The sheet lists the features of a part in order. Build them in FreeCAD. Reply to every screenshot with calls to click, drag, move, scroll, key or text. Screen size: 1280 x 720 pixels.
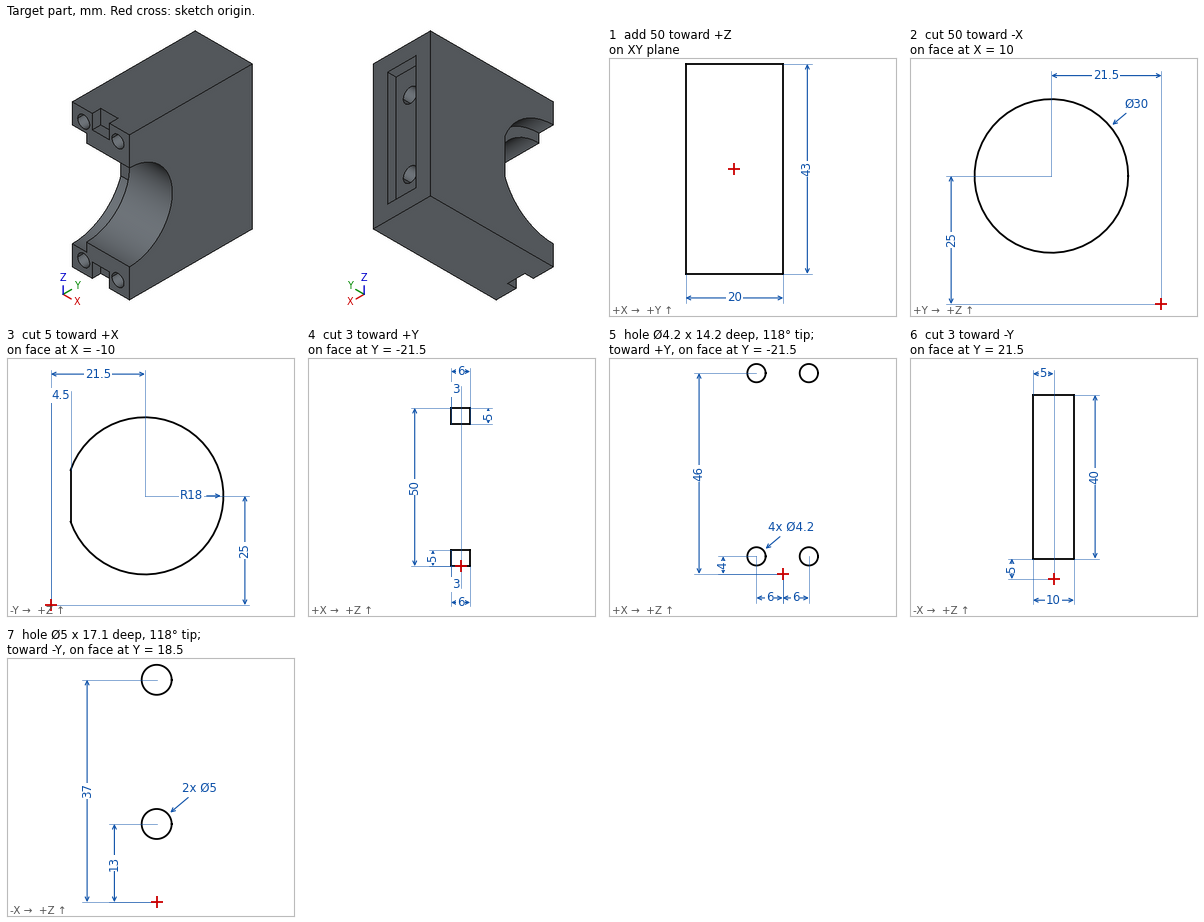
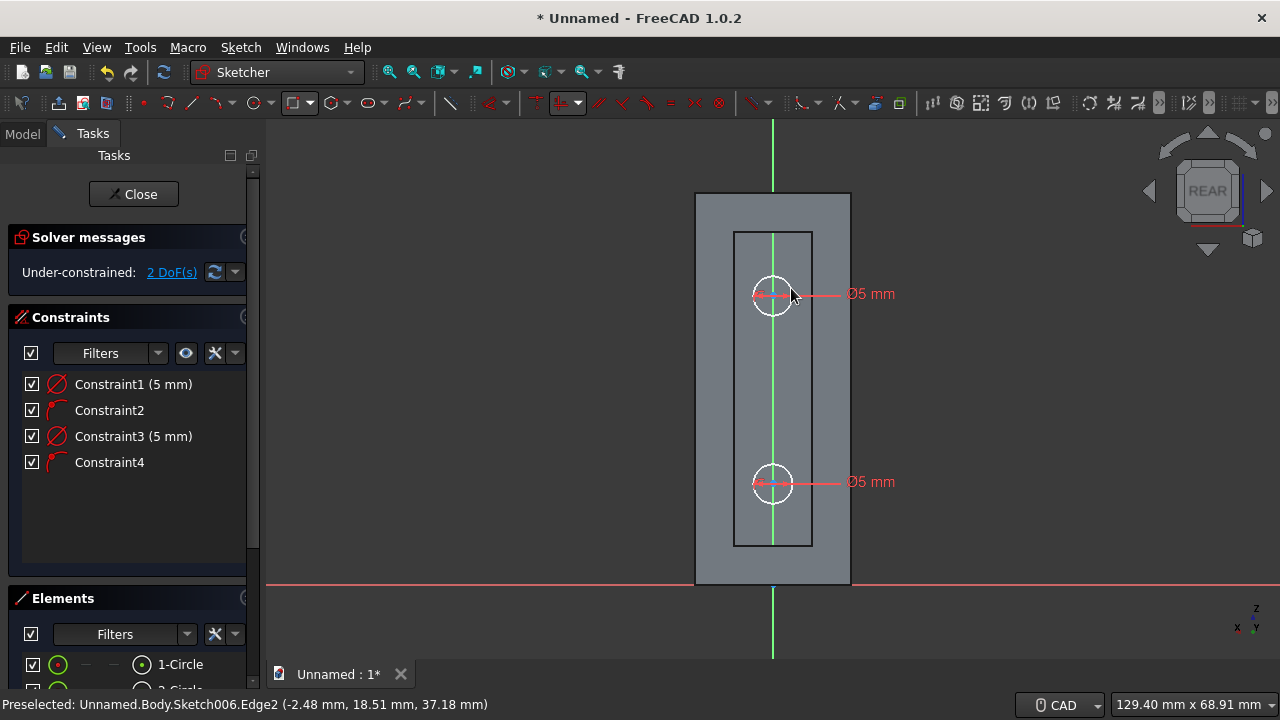
click(490, 104)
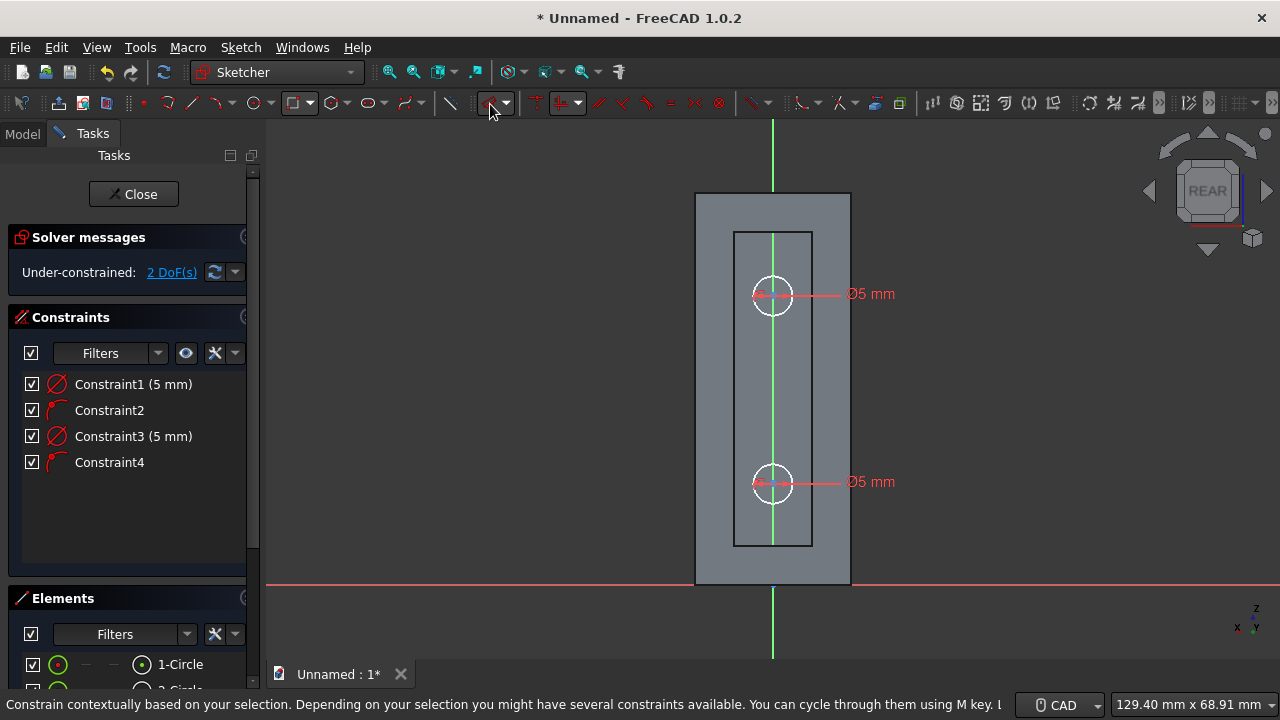
click(773, 484)
click(807, 534)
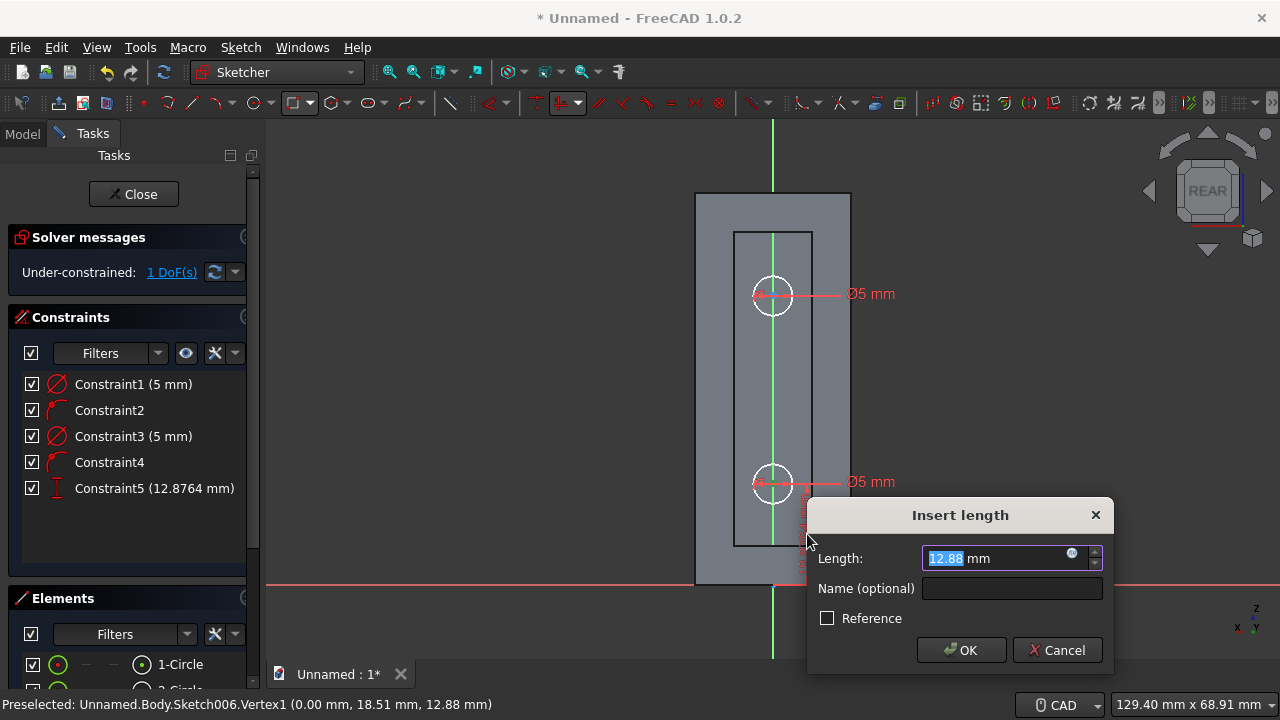
text(13)
key(Return)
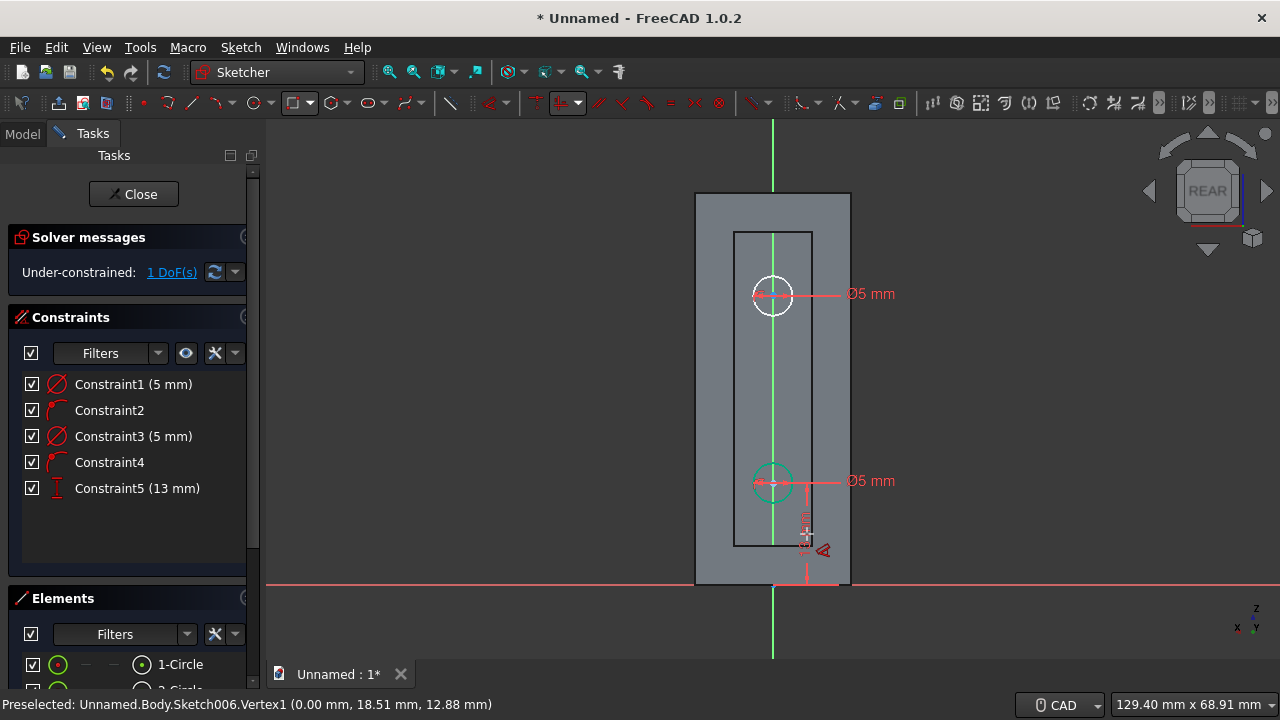
click(773, 296)
click(807, 440)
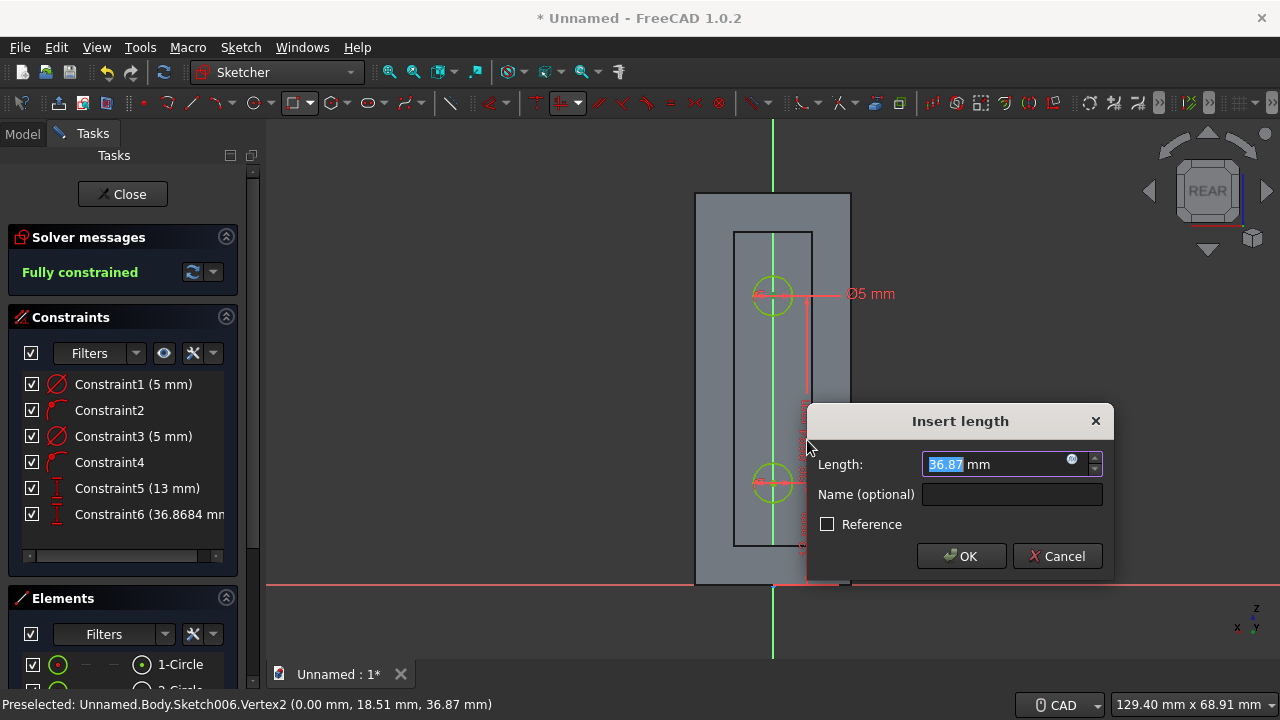
text(37)
key(Return)
key(Escape)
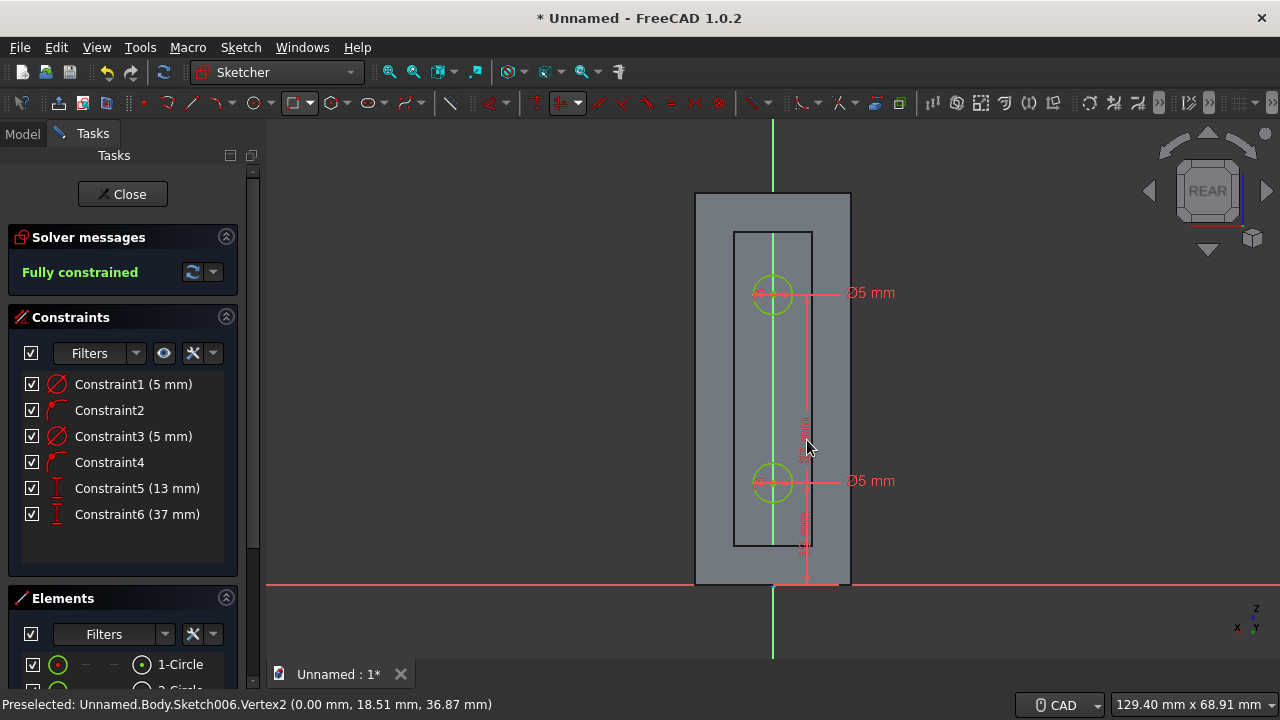
click(123, 194)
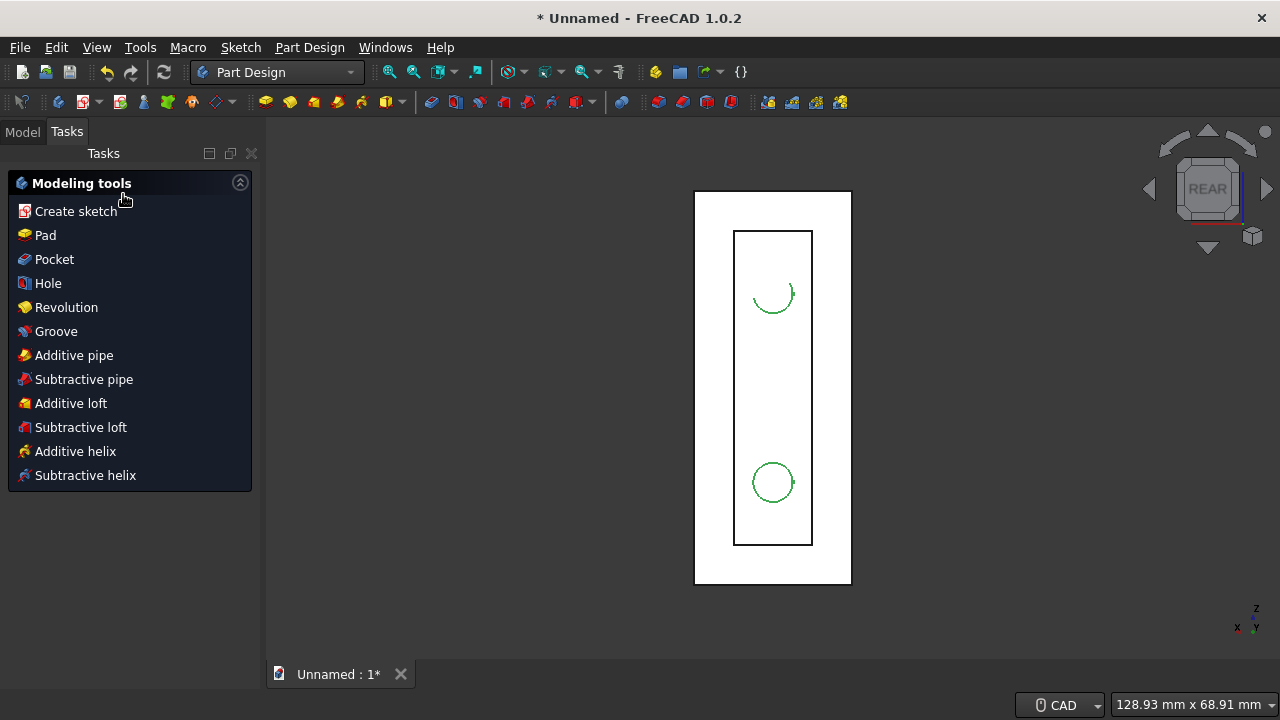
click(456, 102)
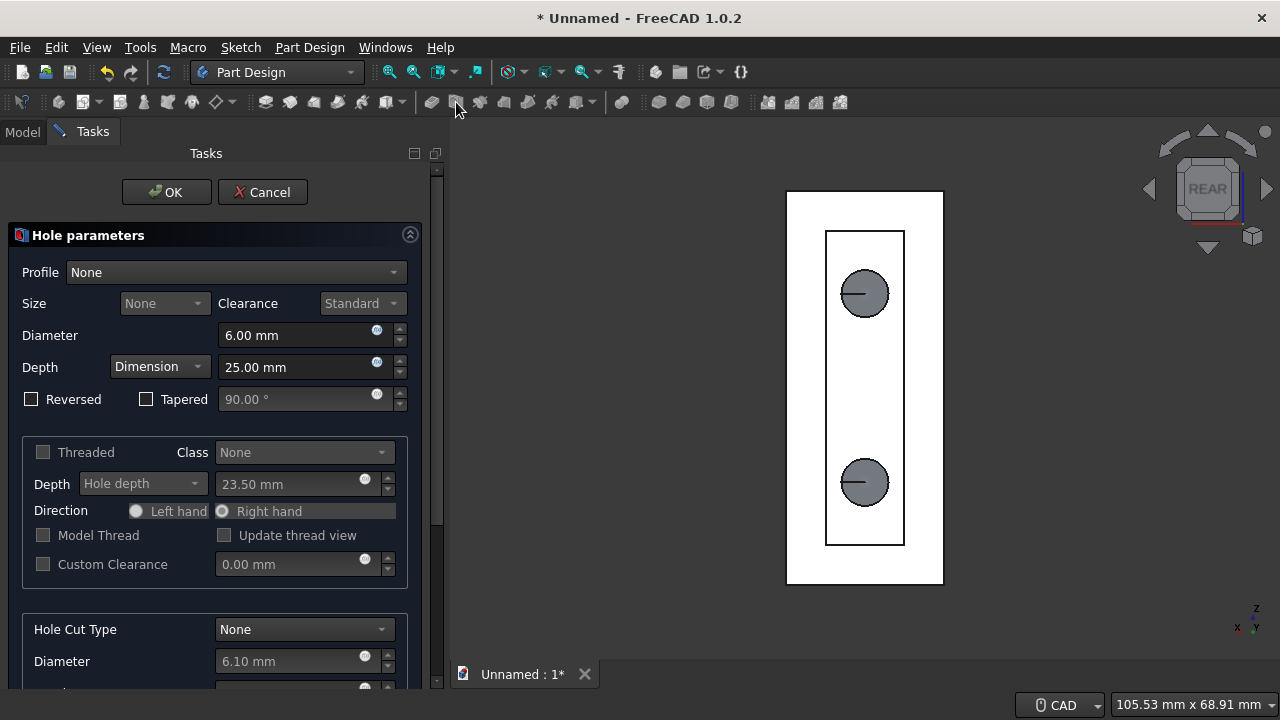
triple_click(305, 335)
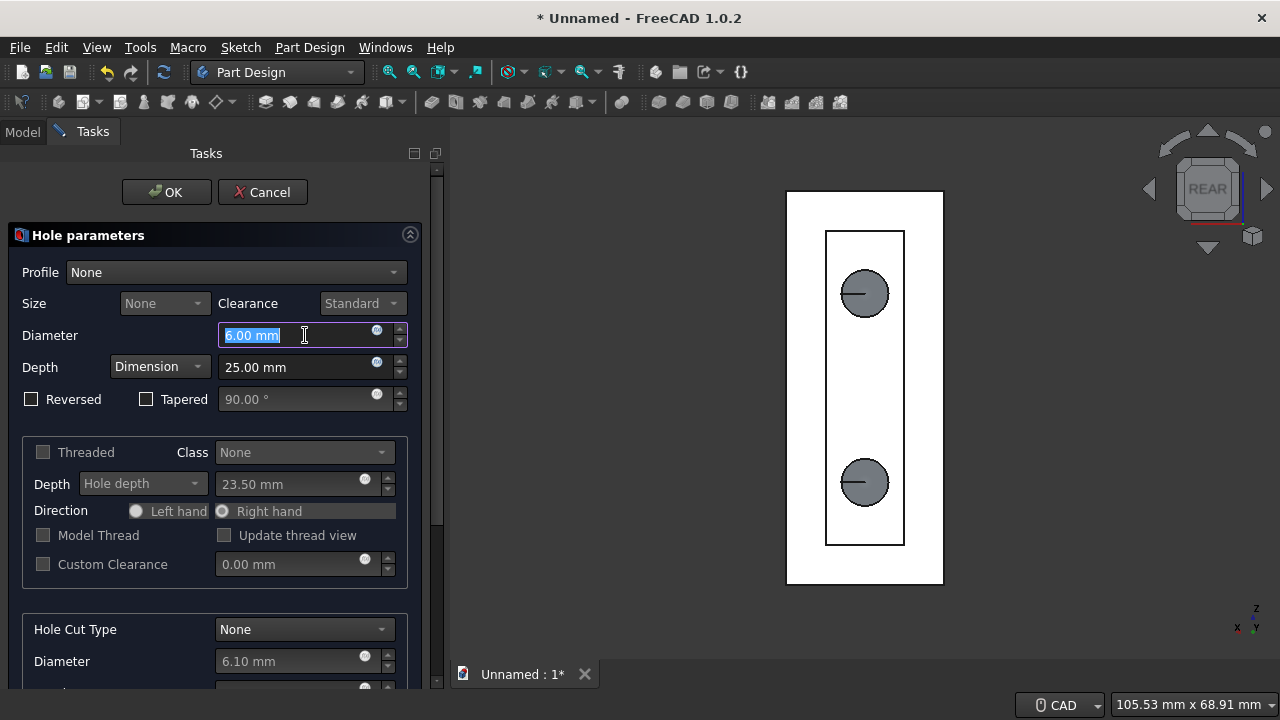
text(5)
key(Tab)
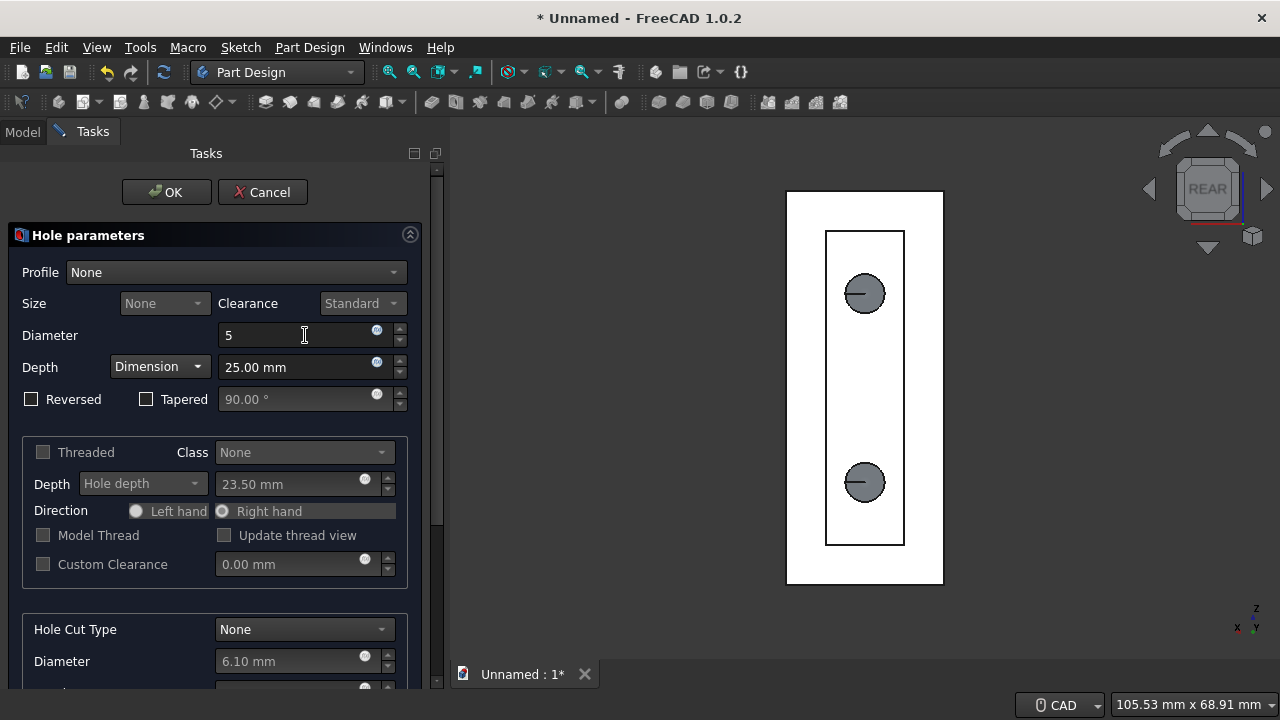
triple_click(305, 367)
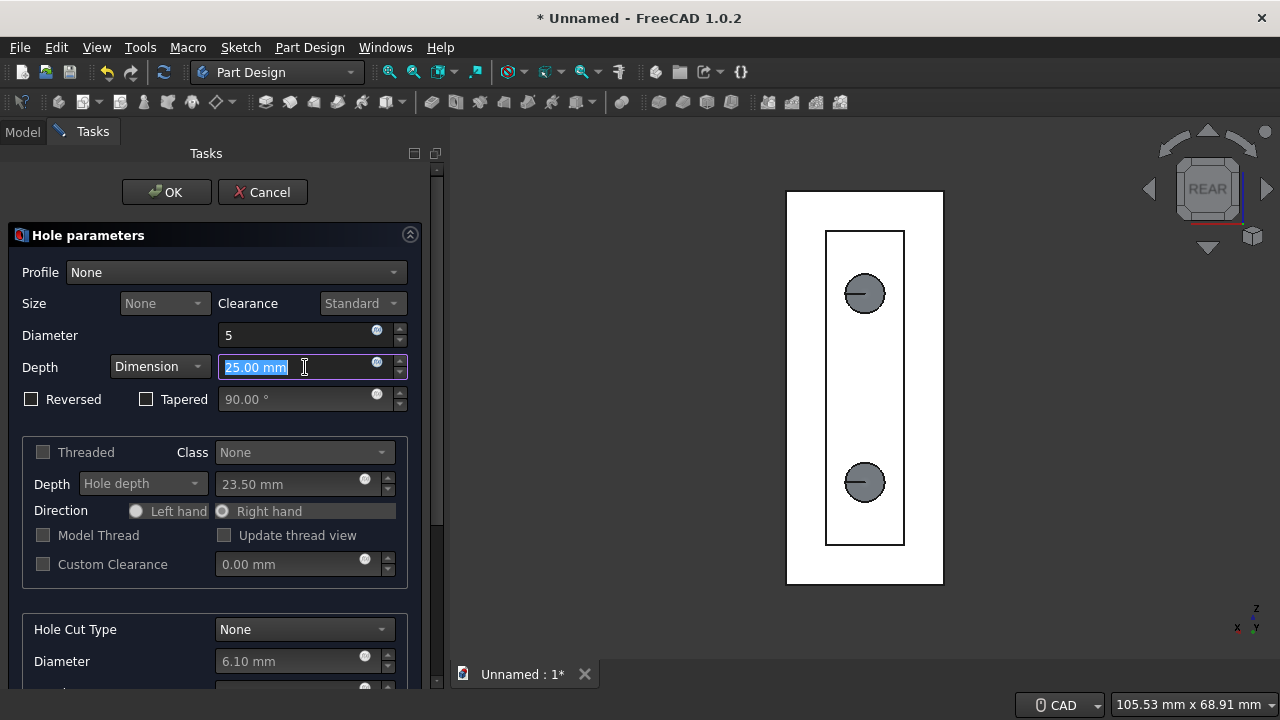
text(17.1)
key(Tab)